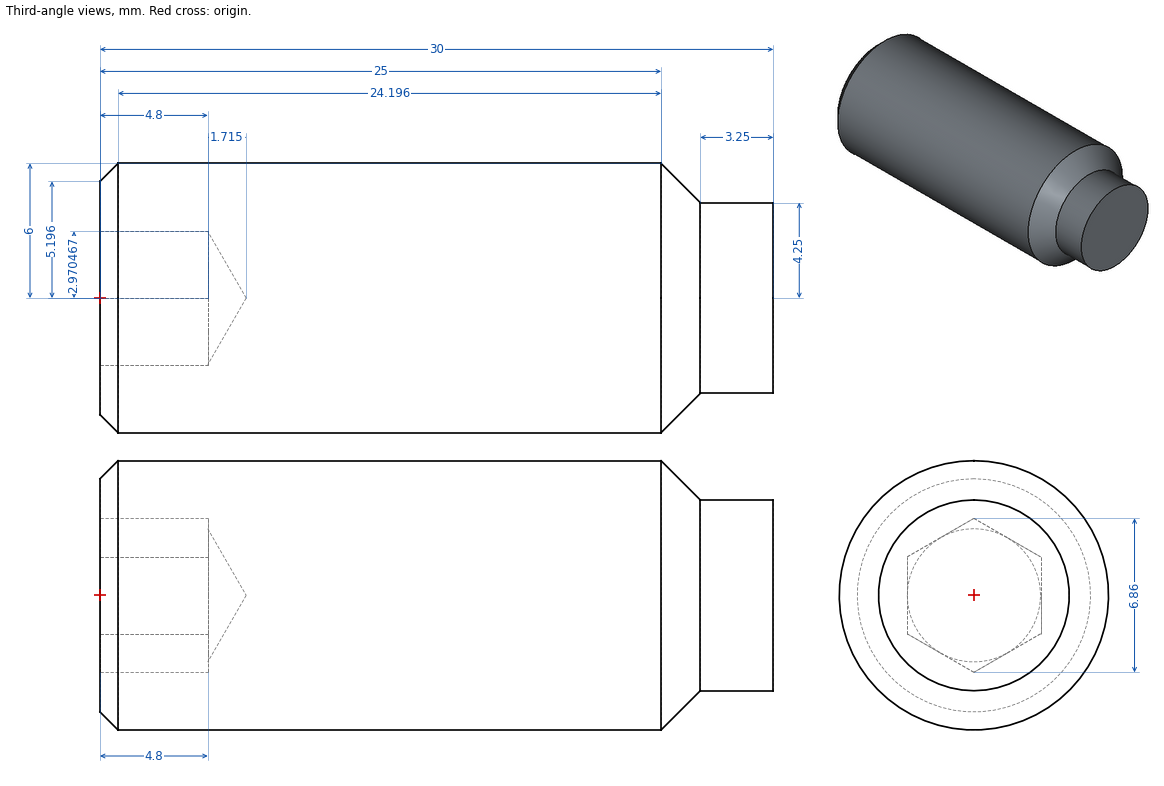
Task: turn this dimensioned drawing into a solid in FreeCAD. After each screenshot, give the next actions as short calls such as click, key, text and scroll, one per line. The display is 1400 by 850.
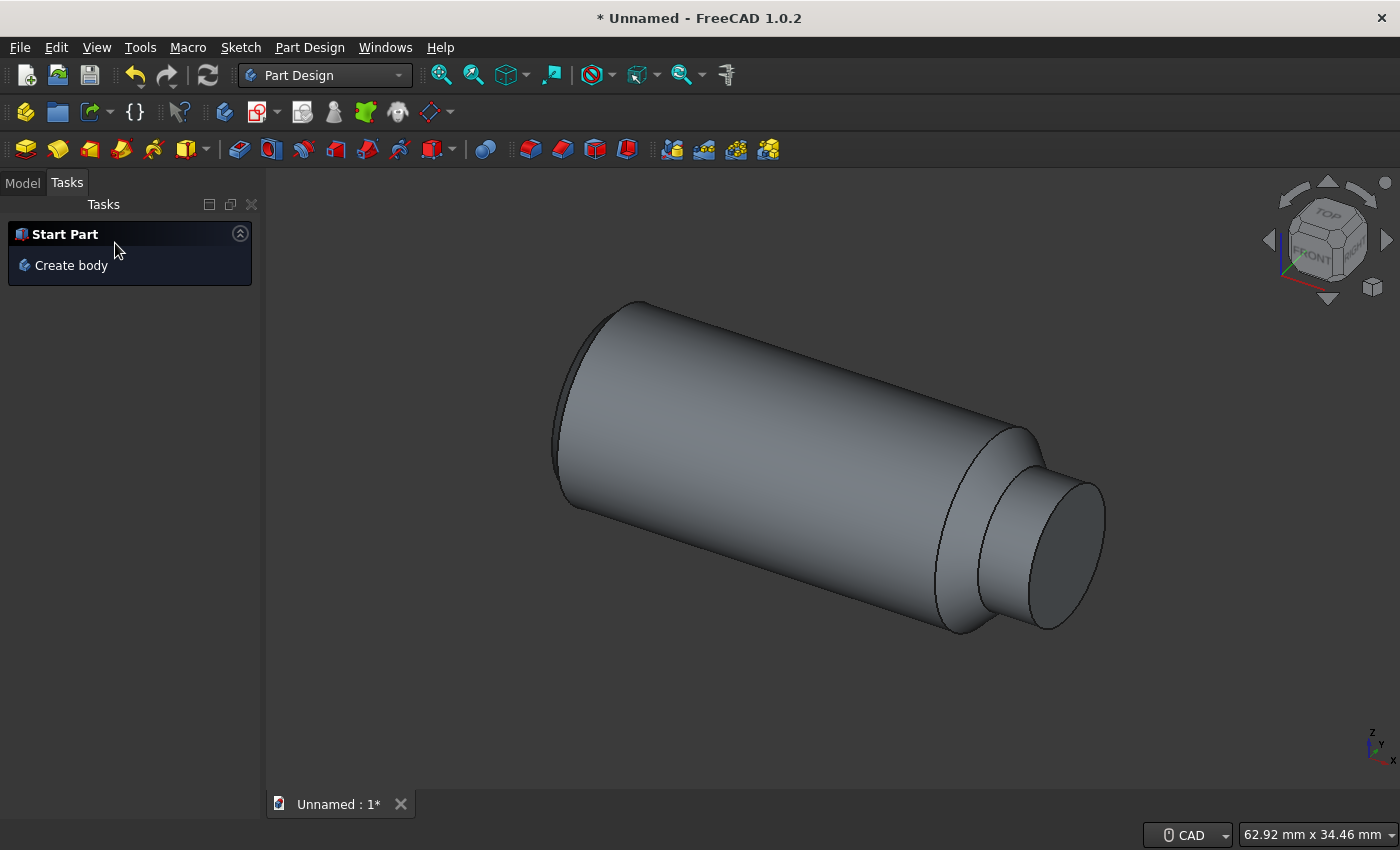
click(258, 112)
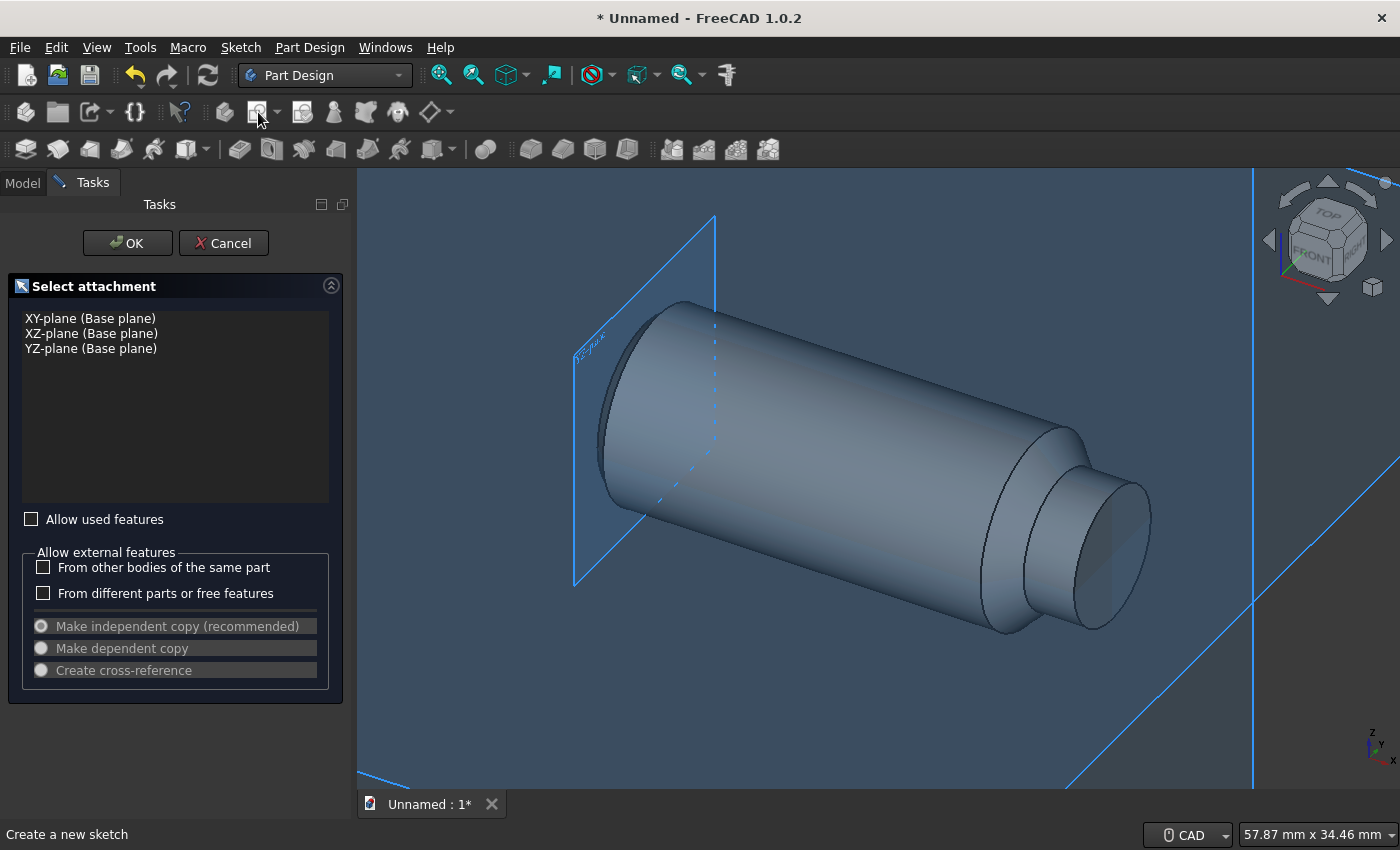
click(82, 318)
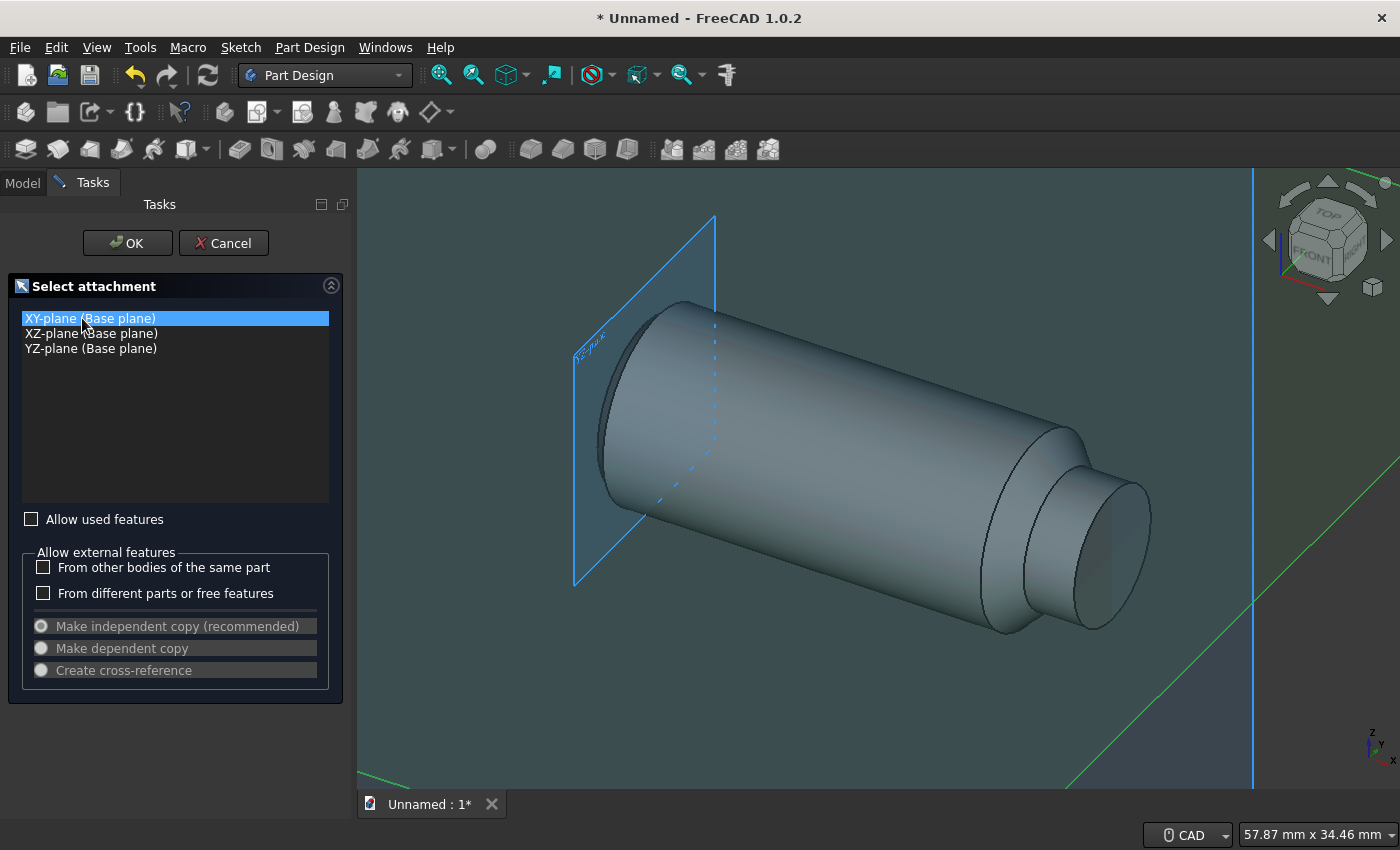
click(128, 243)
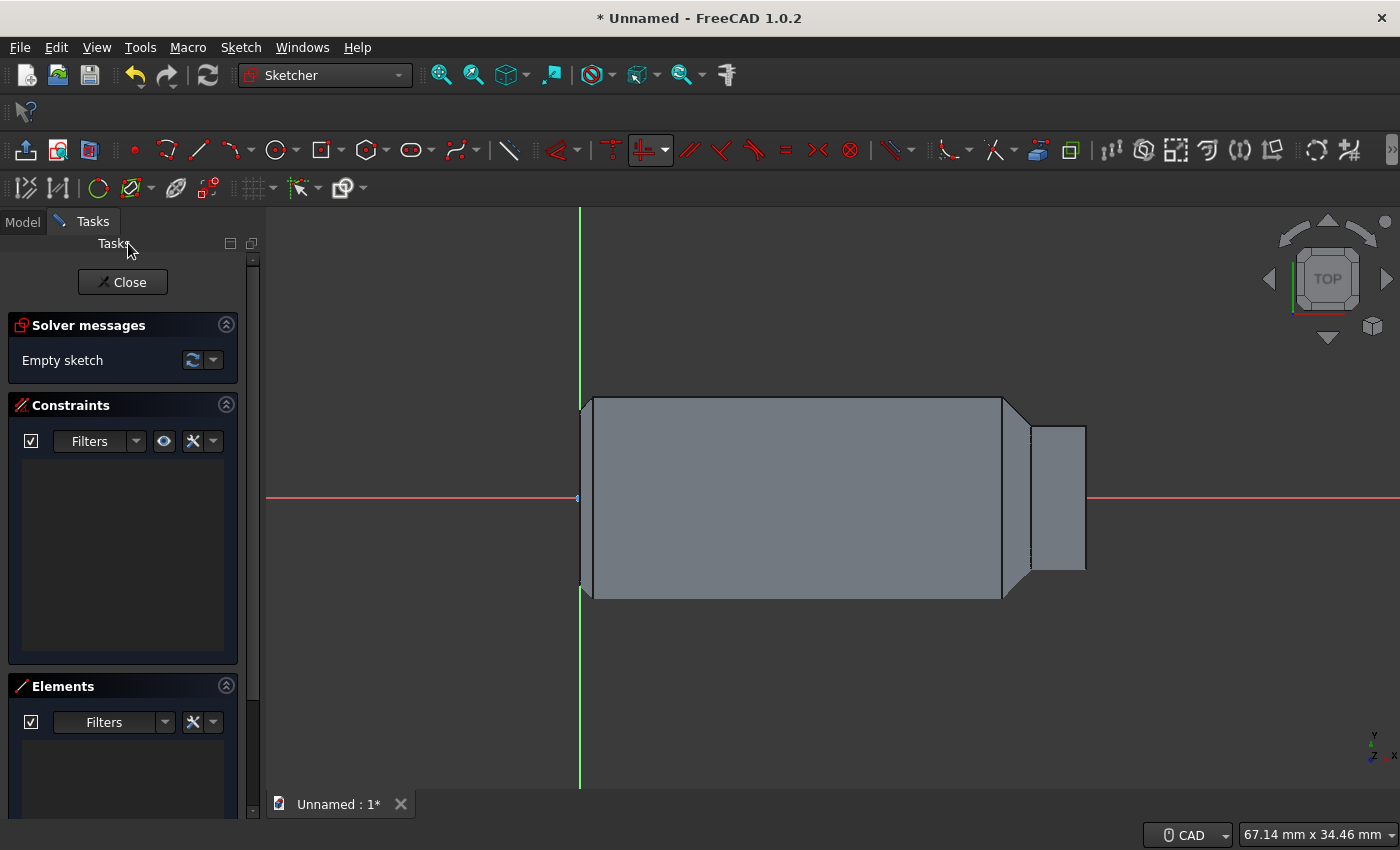
click(90, 150)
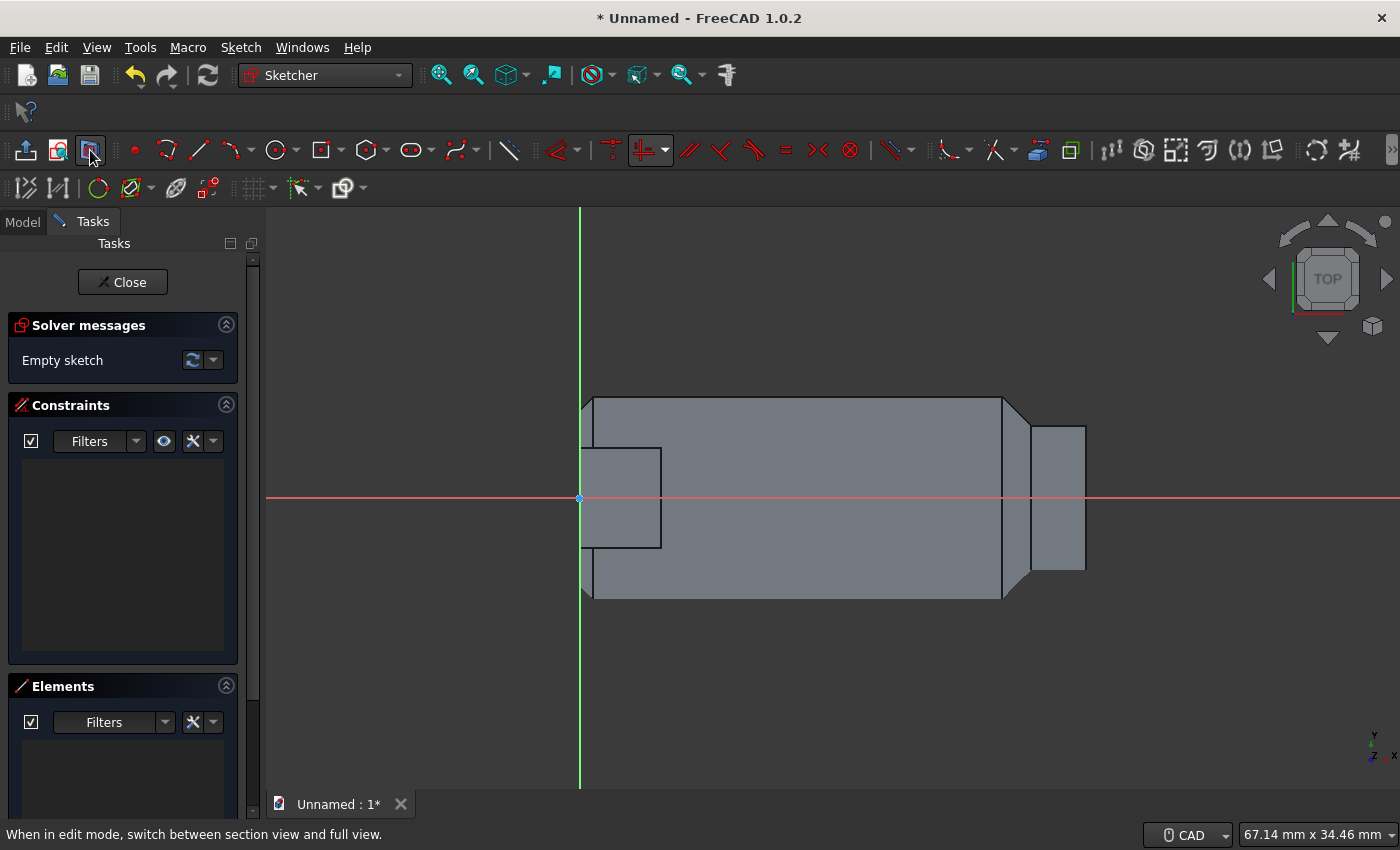
scroll(609, 468, up, 9)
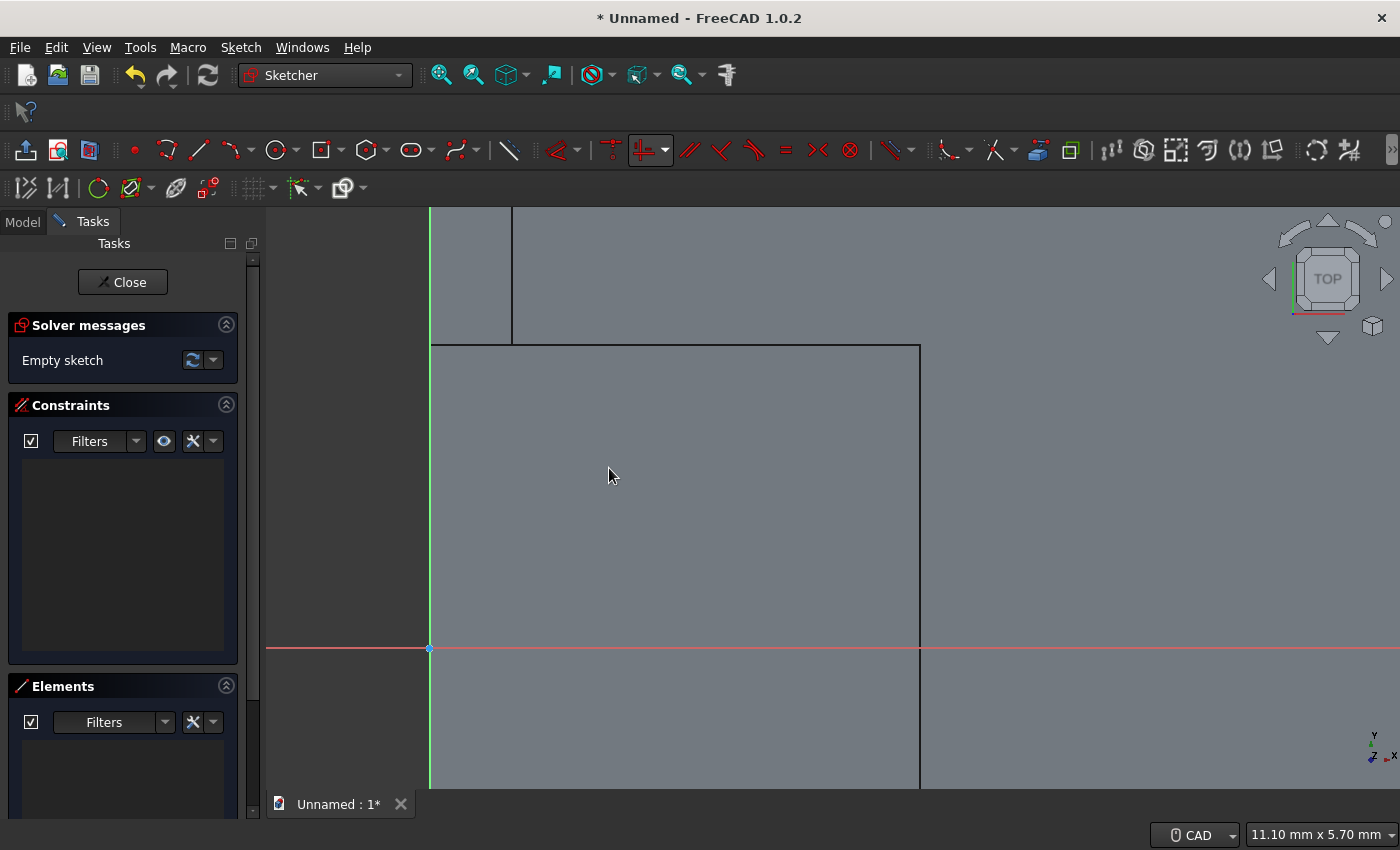
click(168, 150)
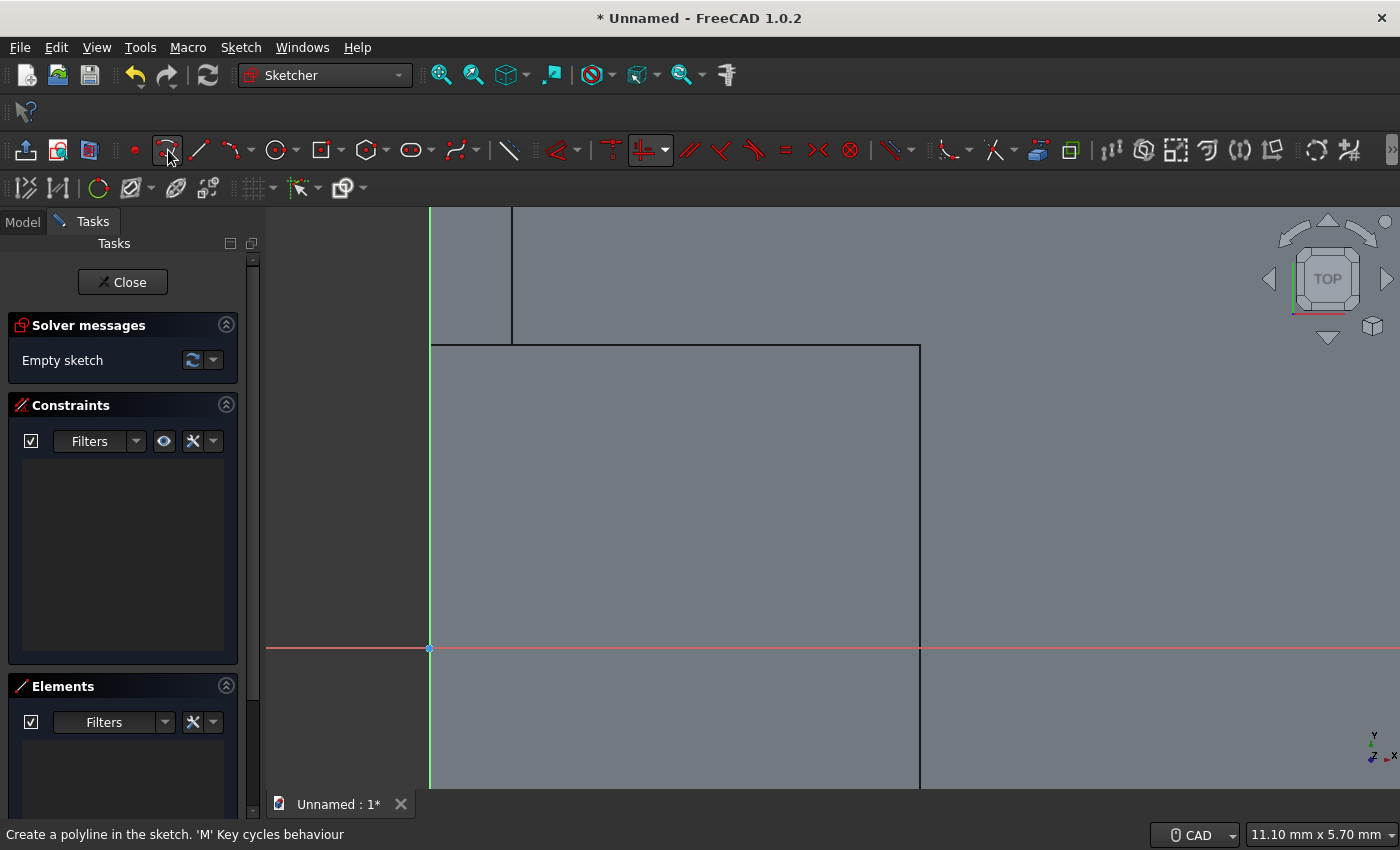
click(920, 648)
click(1096, 639)
click(920, 345)
click(920, 648)
key(Escape)
key(Escape)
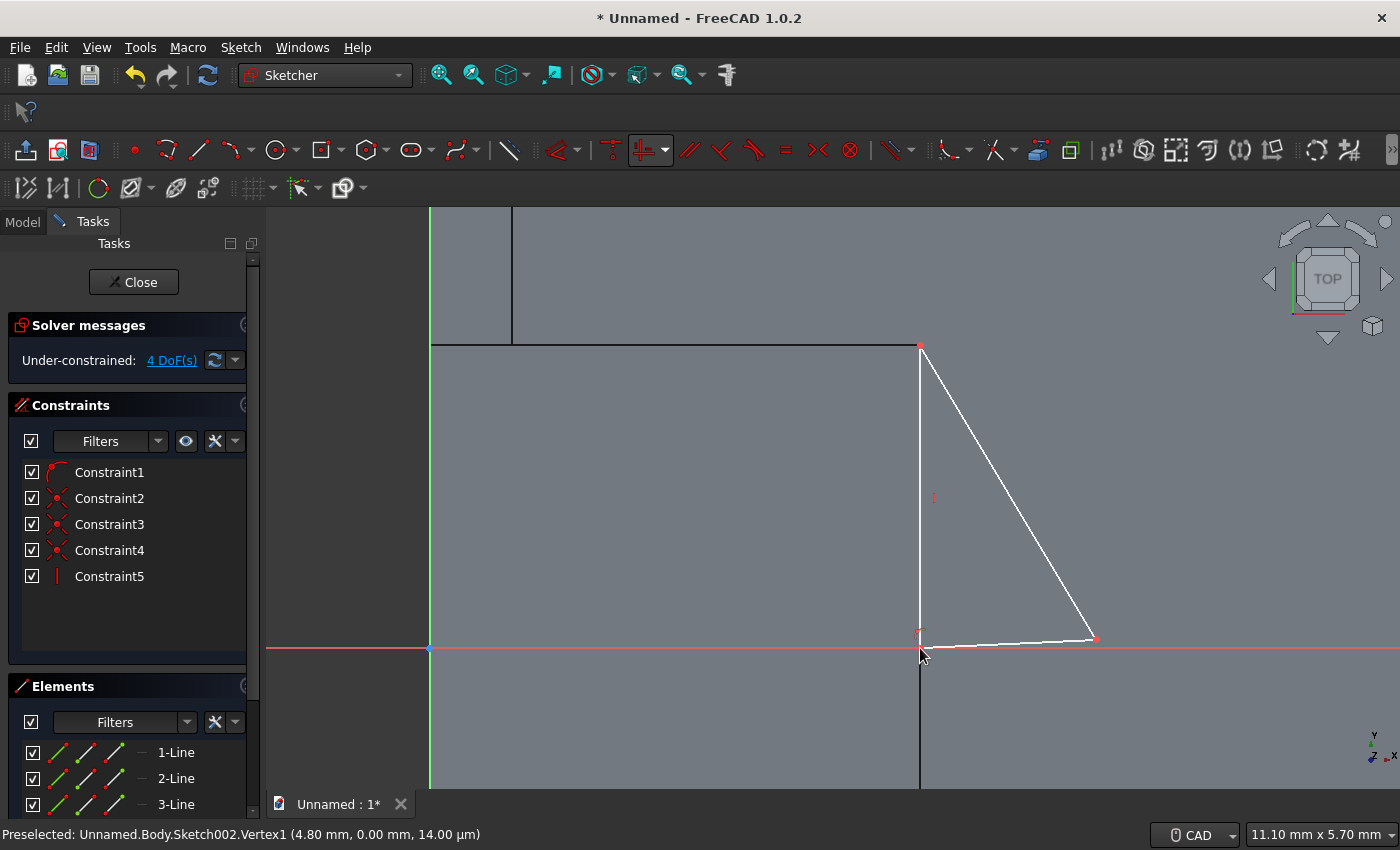
click(973, 646)